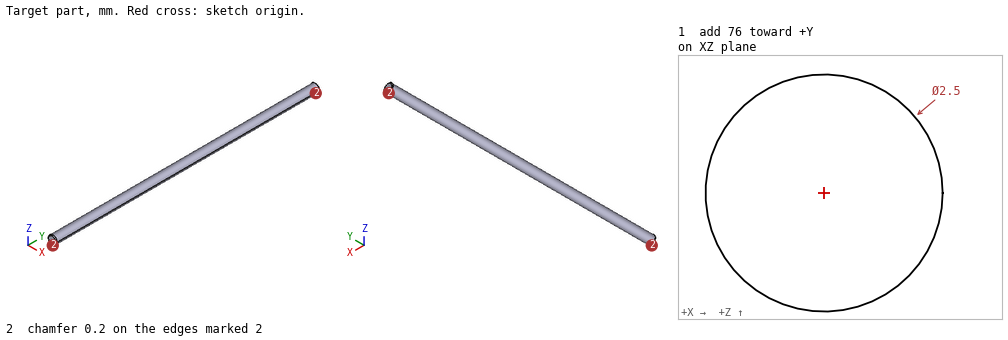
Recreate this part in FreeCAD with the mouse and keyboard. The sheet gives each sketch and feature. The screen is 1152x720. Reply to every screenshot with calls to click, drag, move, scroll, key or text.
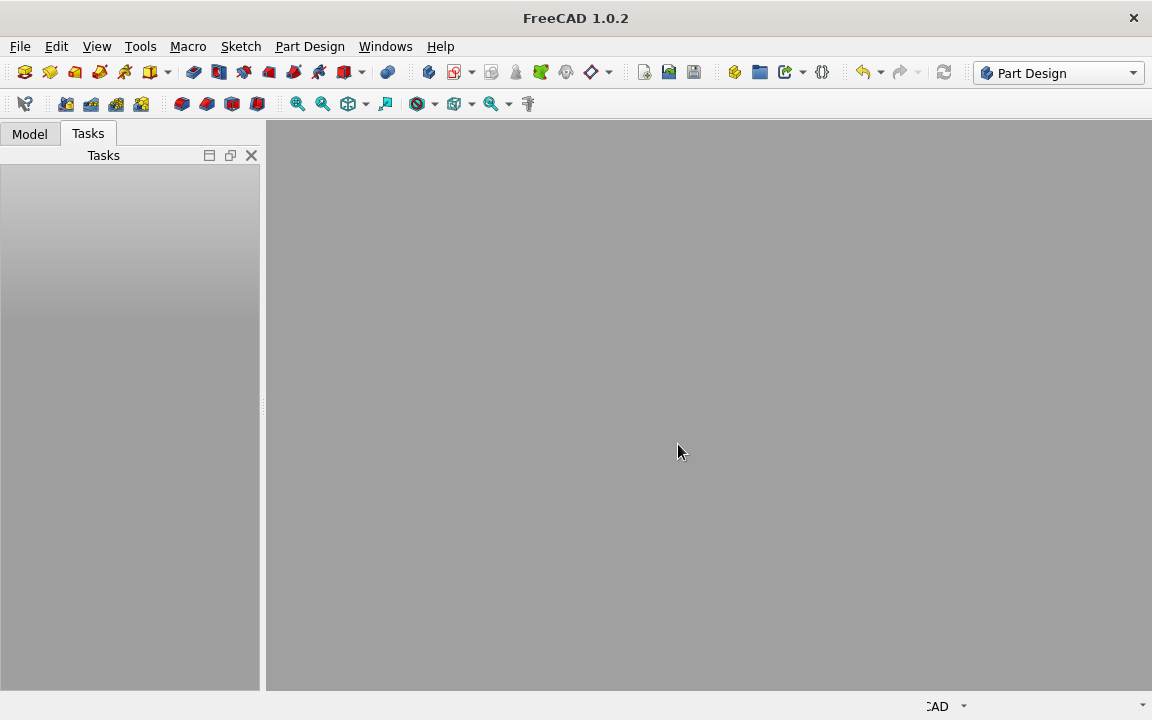
click(644, 72)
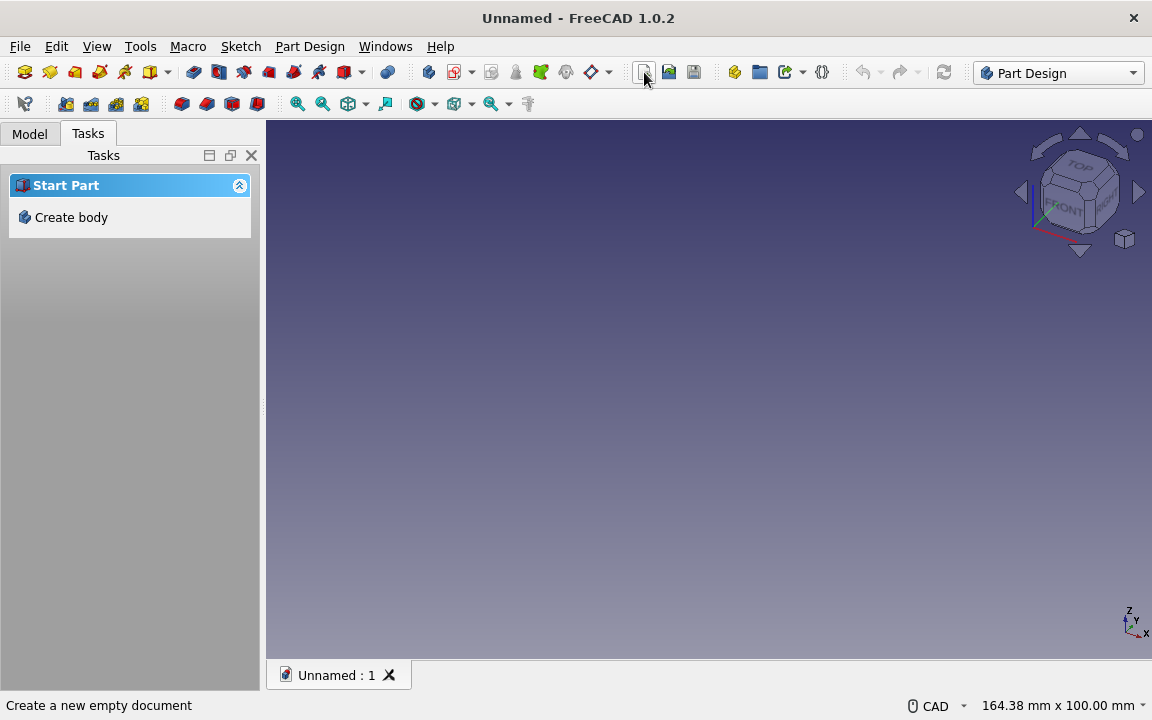
click(454, 72)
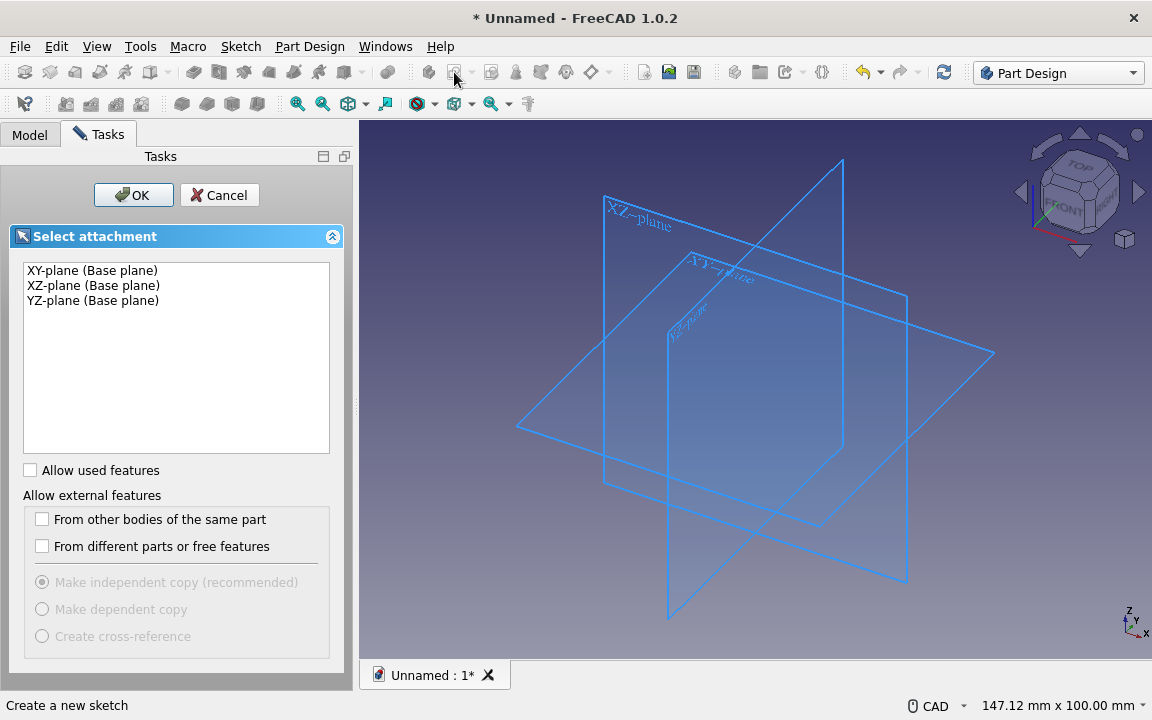
click(84, 286)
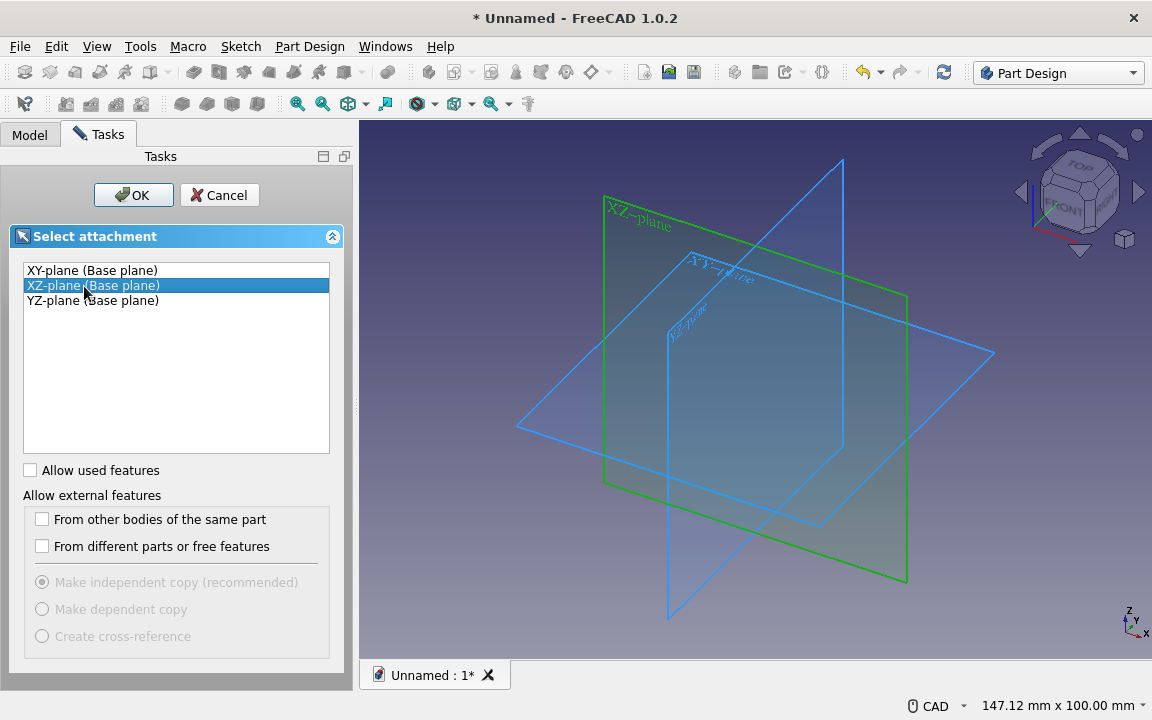
click(134, 195)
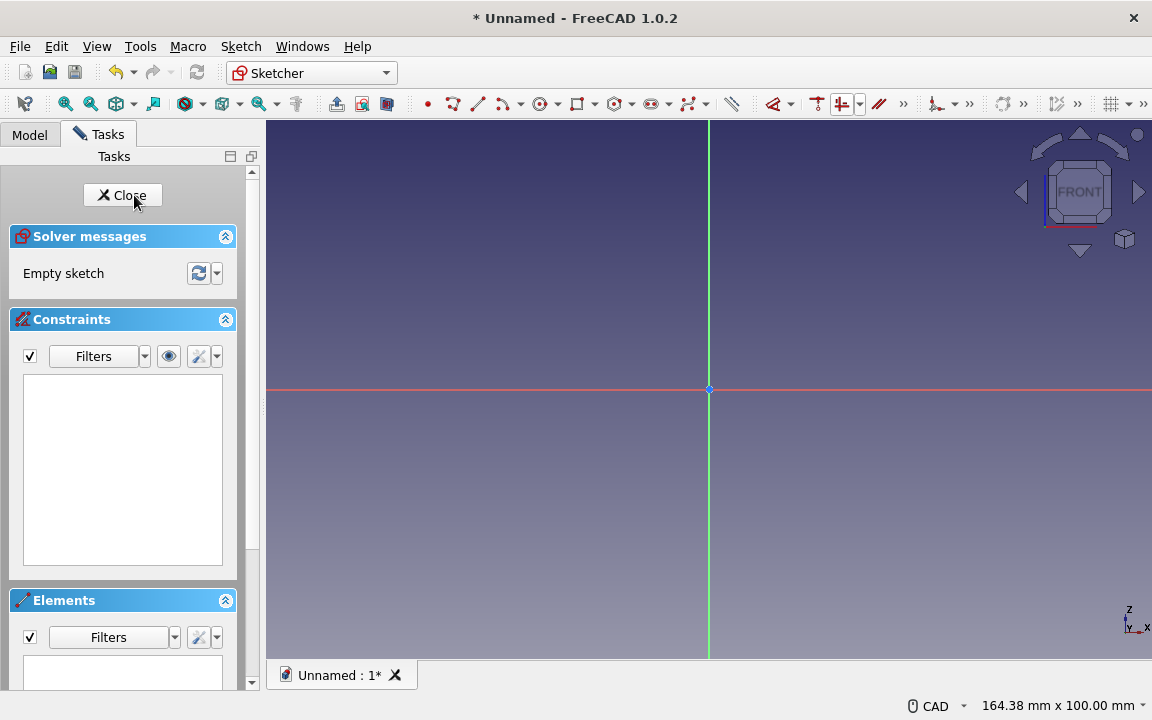
scroll(713, 390, up, 15)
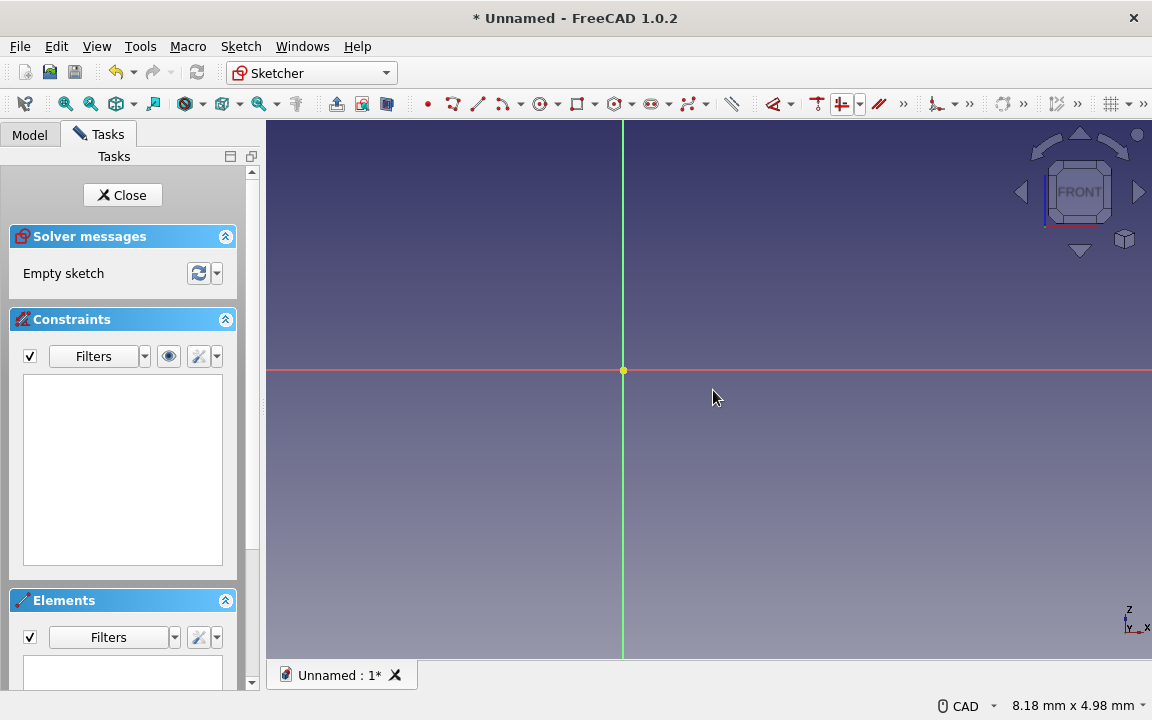
click(540, 104)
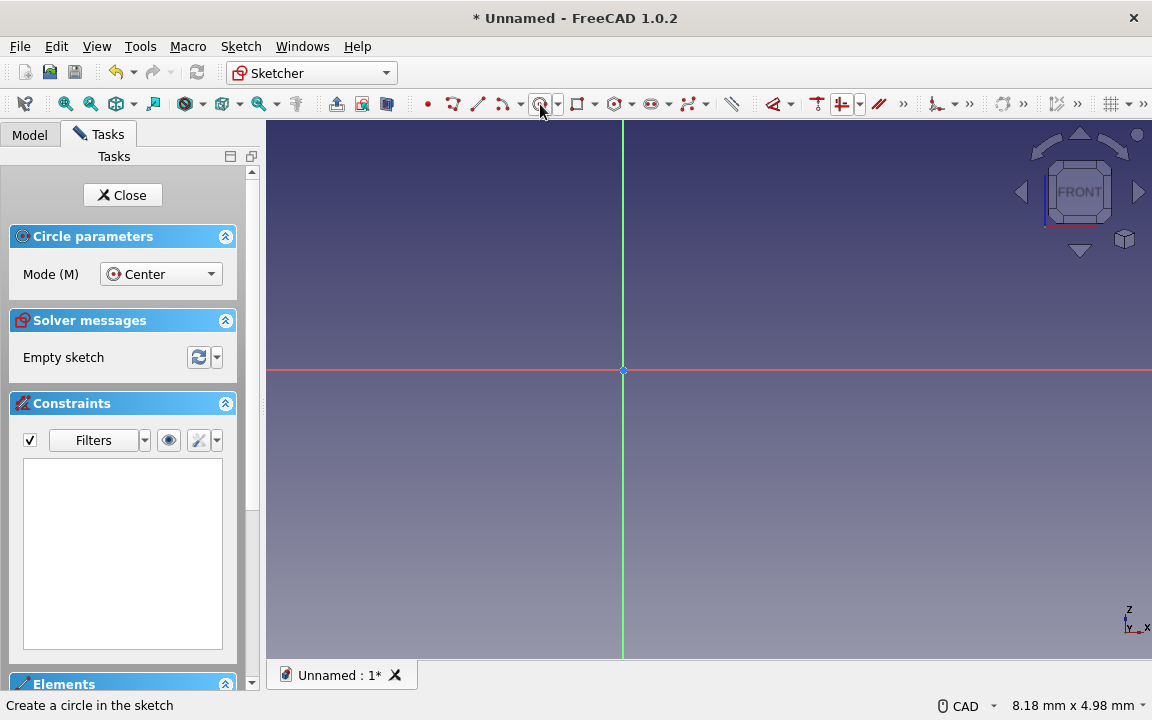
click(623, 370)
click(719, 275)
key(Escape)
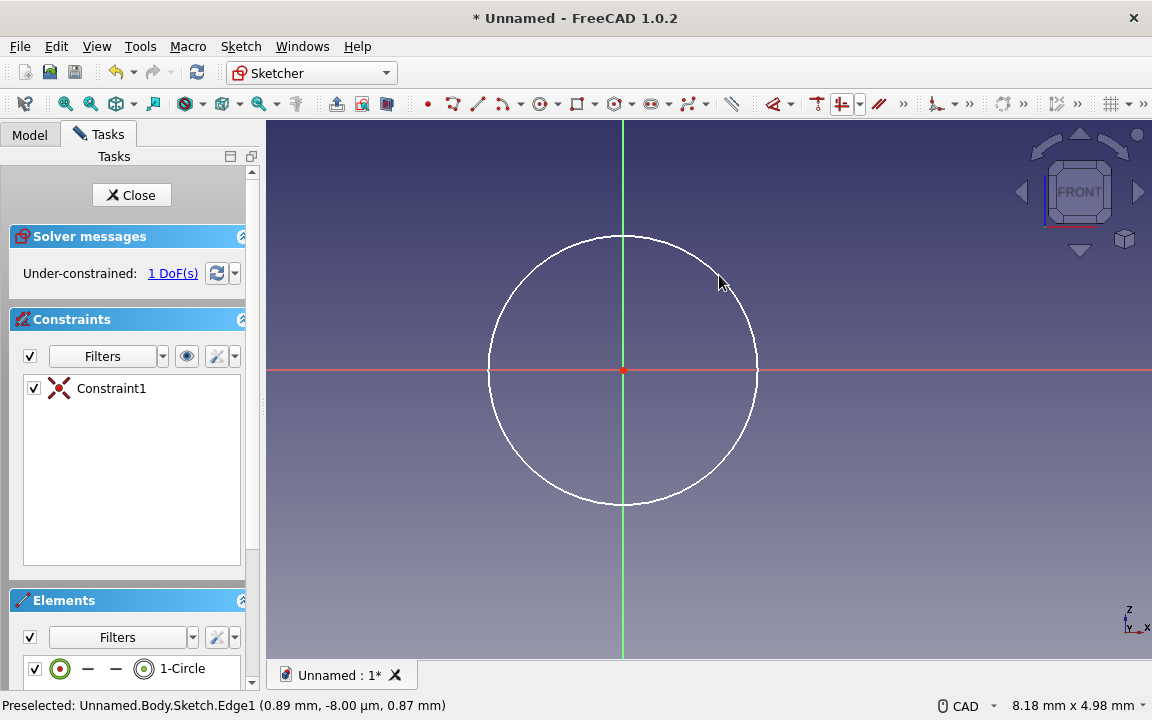
click(772, 104)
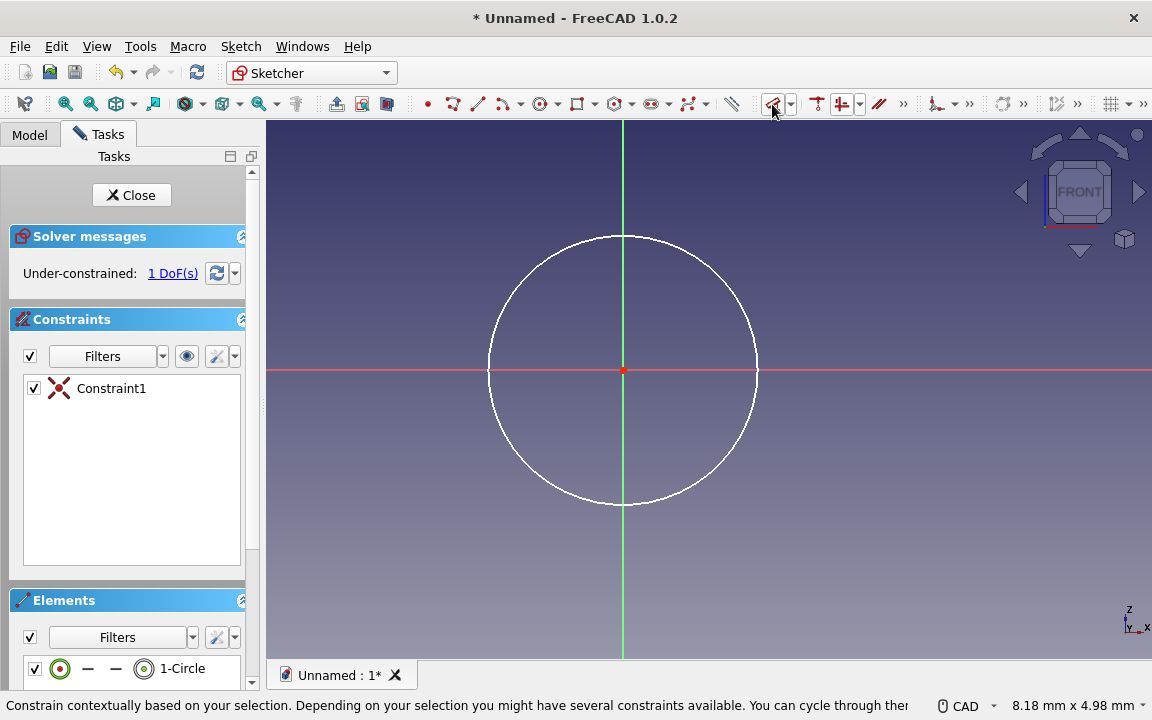
click(718, 275)
click(741, 252)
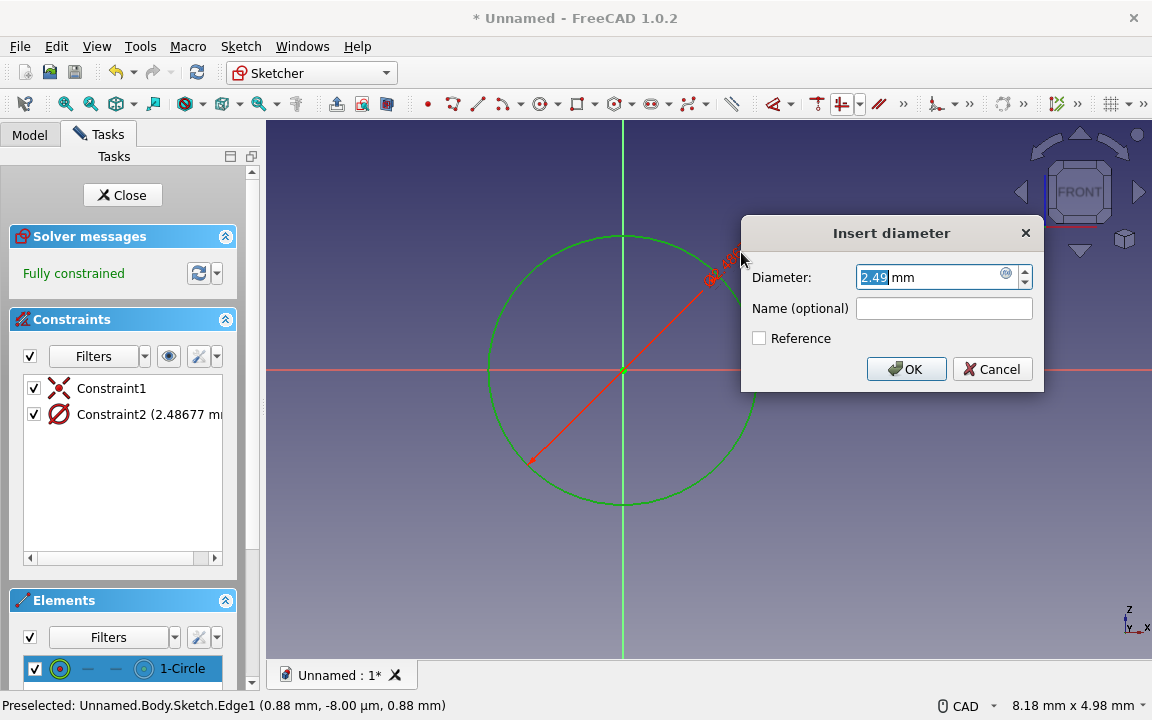
text(2.5)
key(Return)
key(Escape)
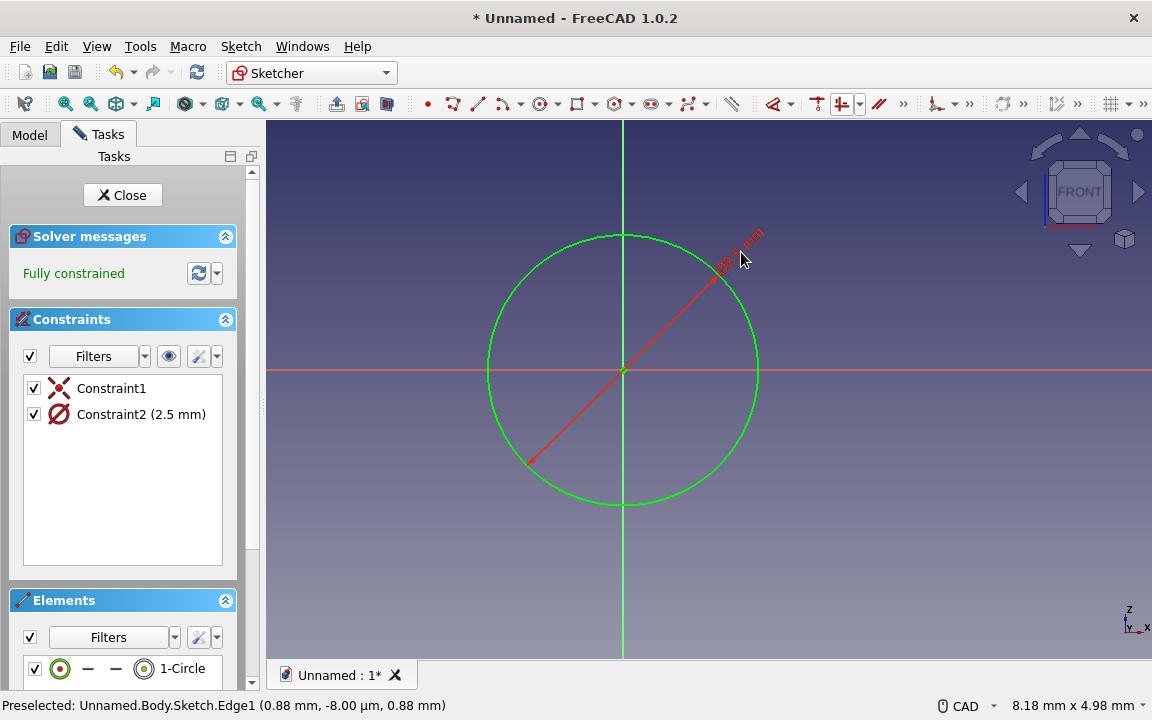
click(123, 195)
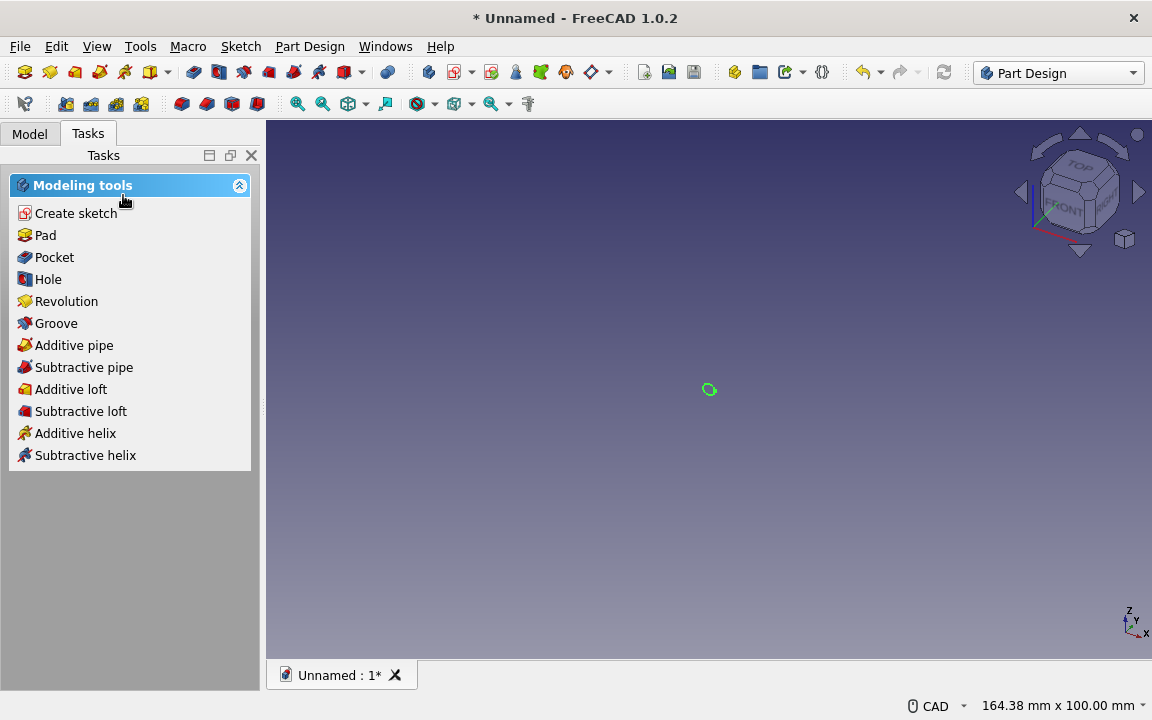
click(25, 72)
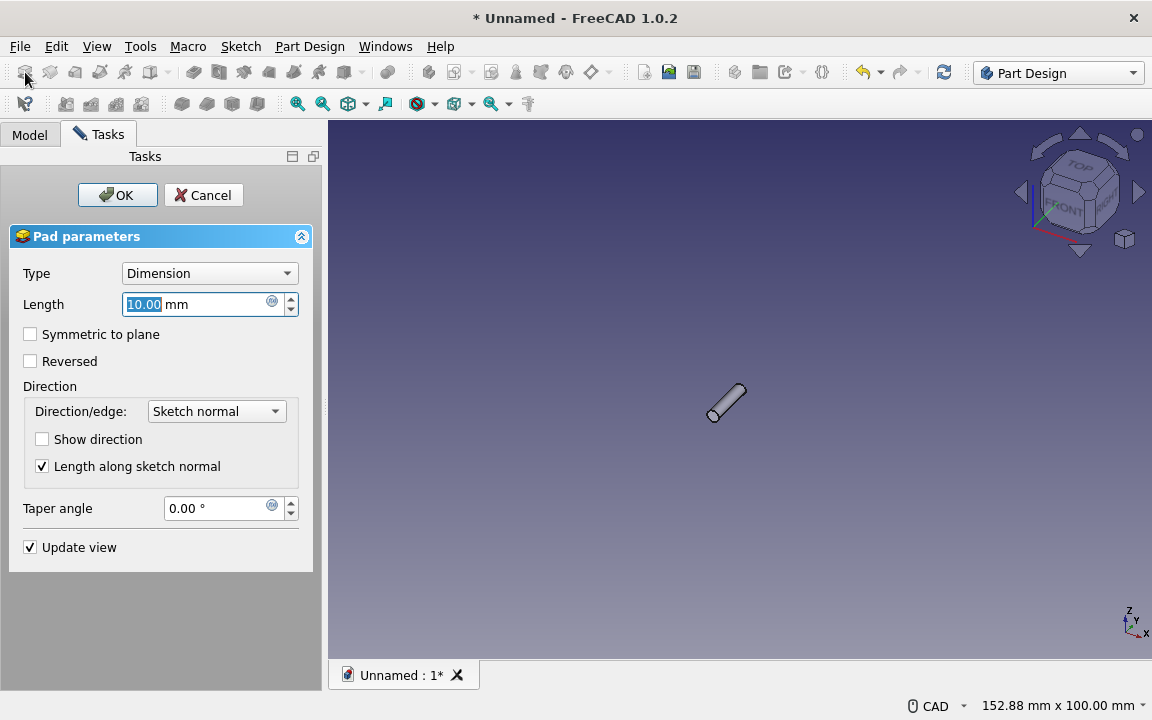
text(76)
key(Tab)